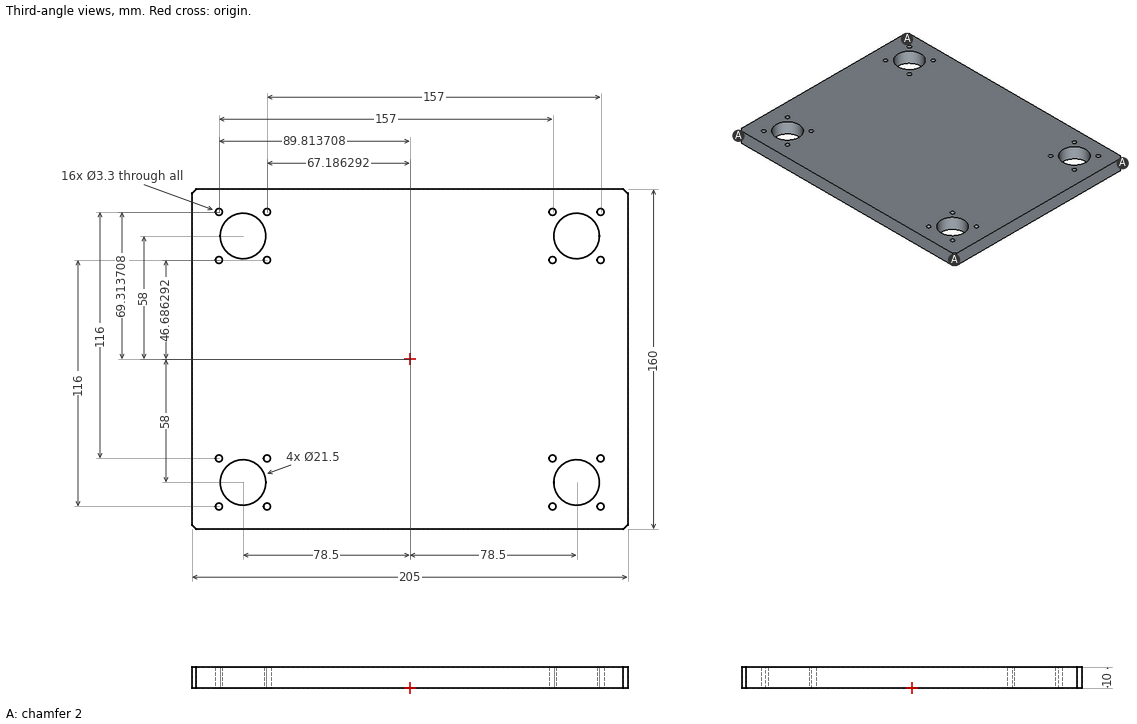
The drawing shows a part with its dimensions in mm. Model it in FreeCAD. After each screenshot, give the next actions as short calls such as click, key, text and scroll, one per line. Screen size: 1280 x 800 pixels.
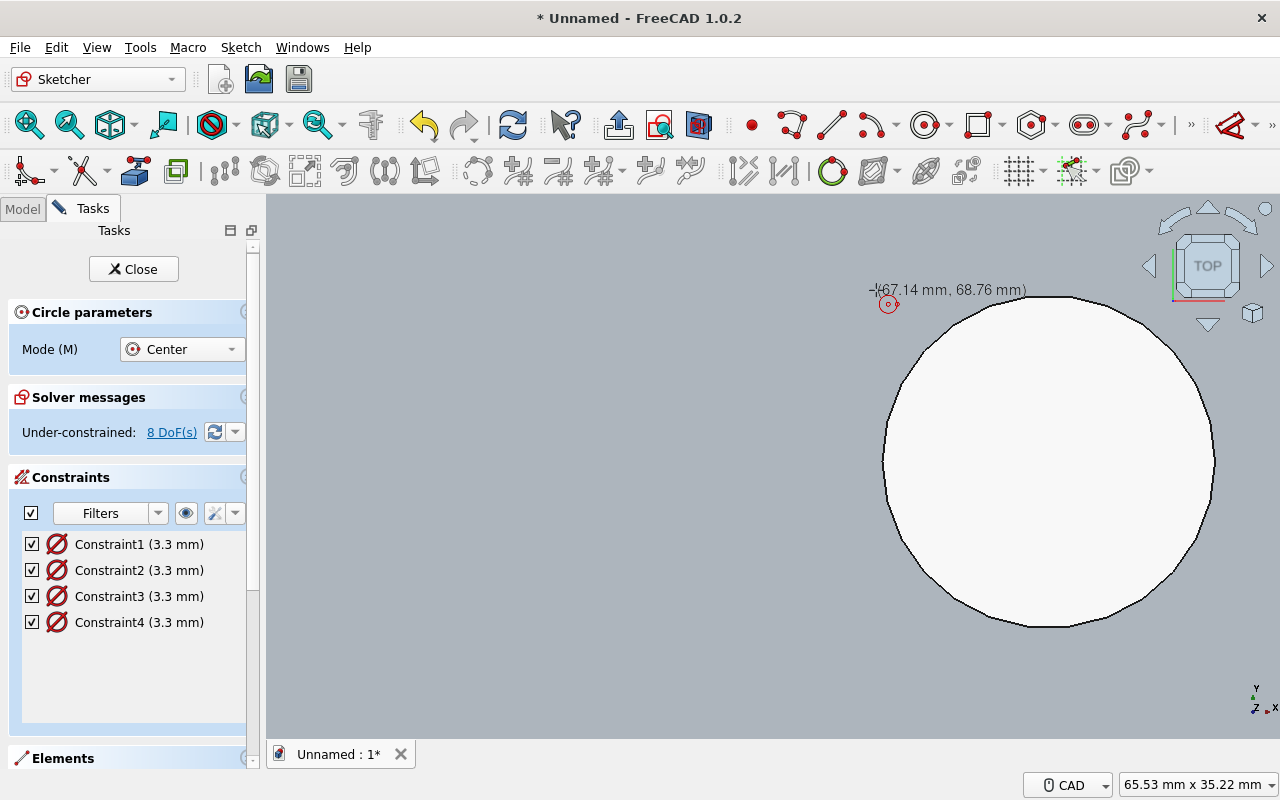
scroll(877, 290, down, 9)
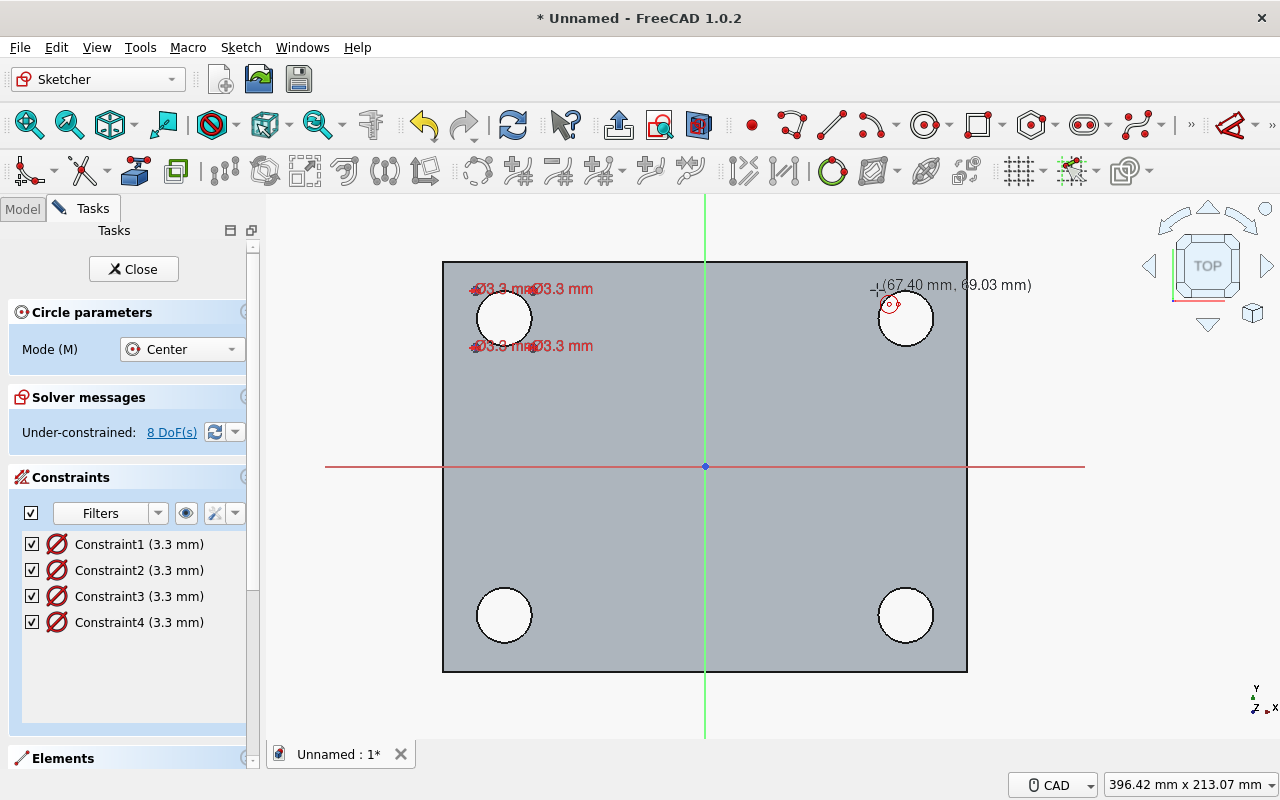
click(877, 290)
move(880, 287)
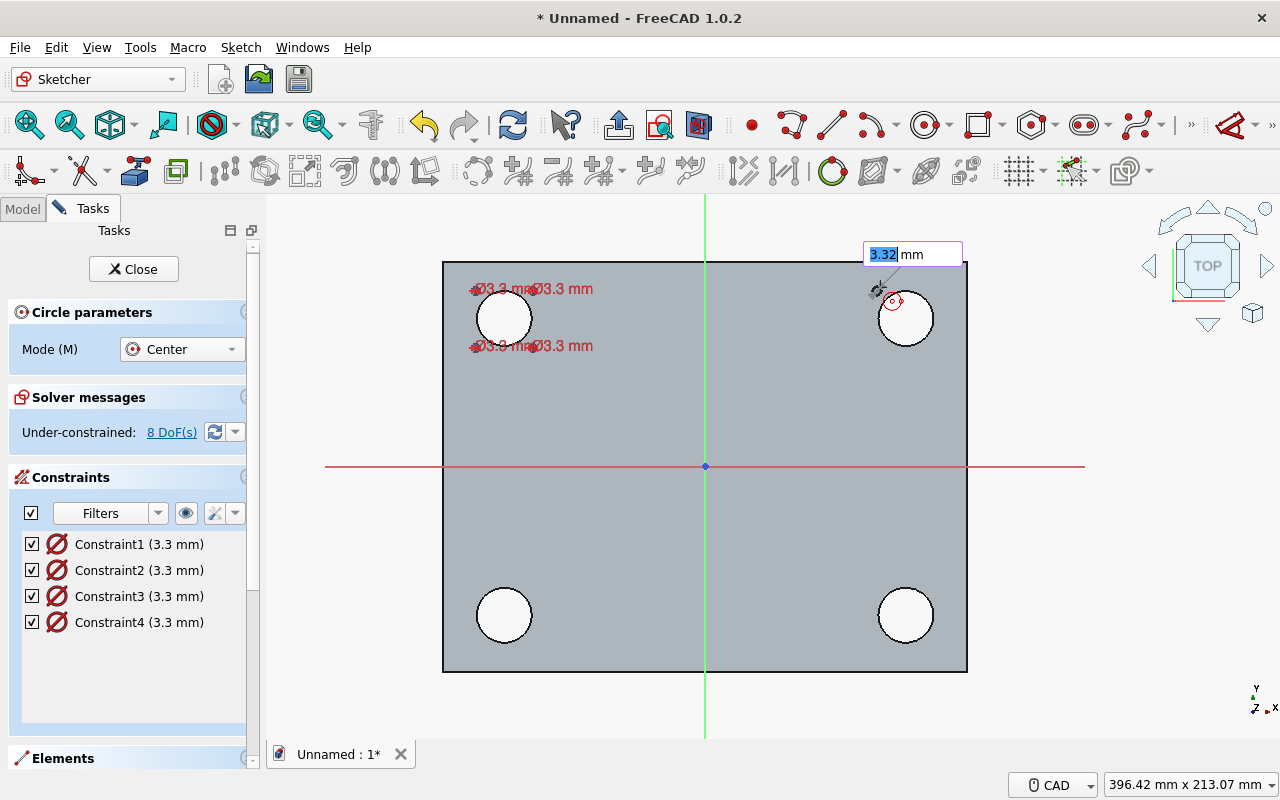
text(3.3)
key(Return)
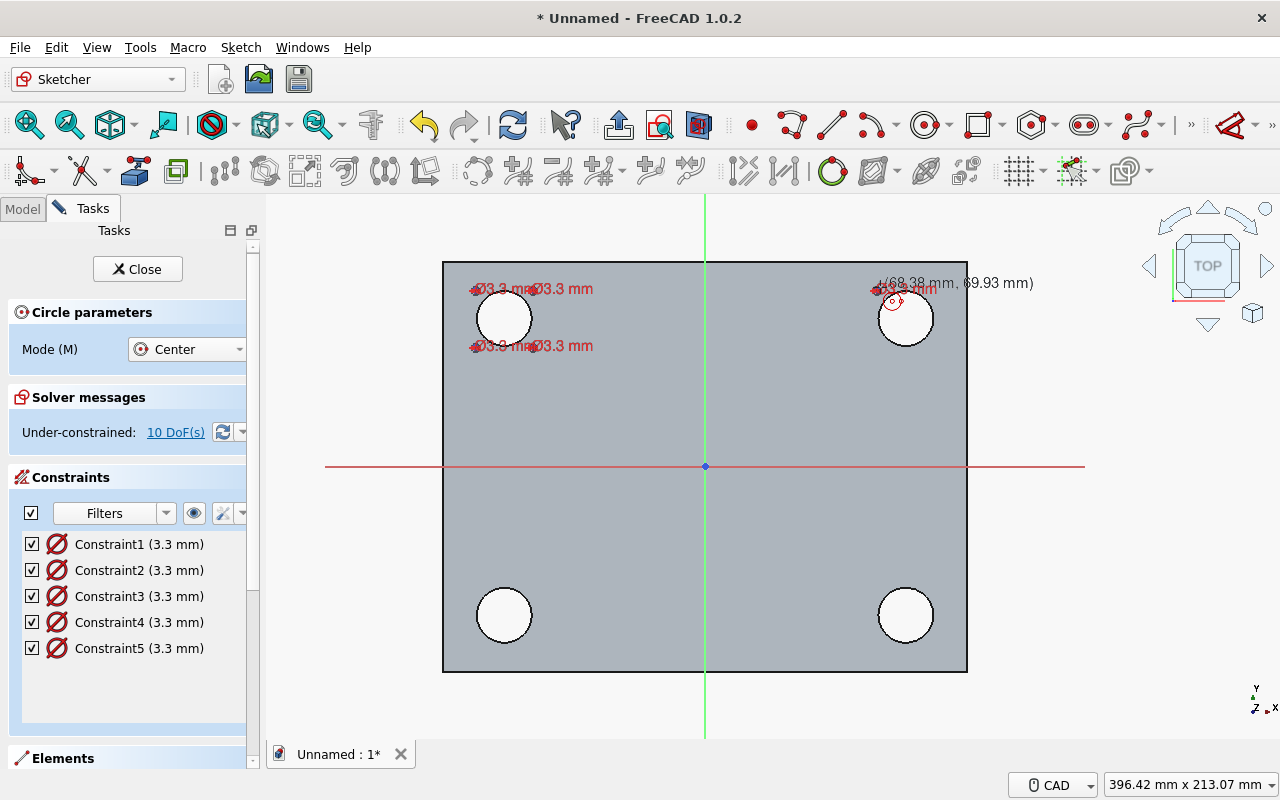
scroll(935, 290, up, 9)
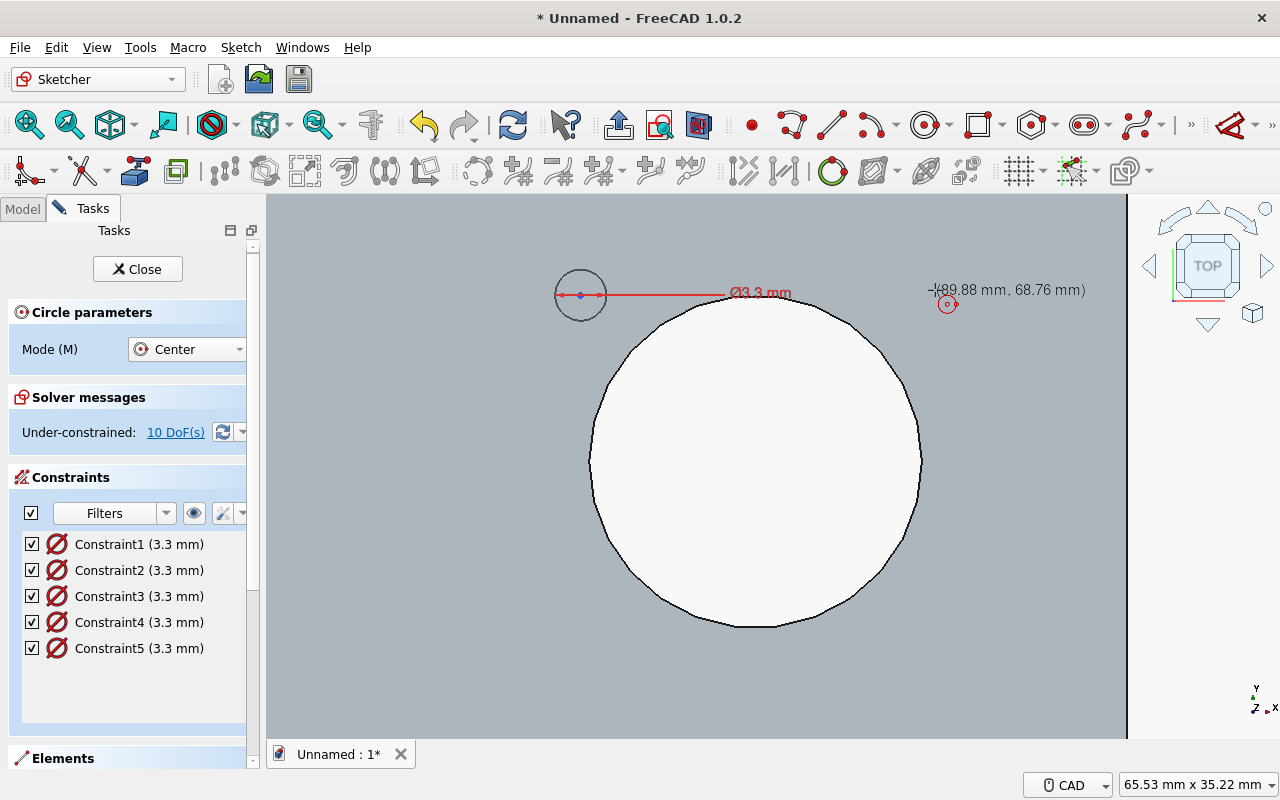
scroll(935, 290, down, 9)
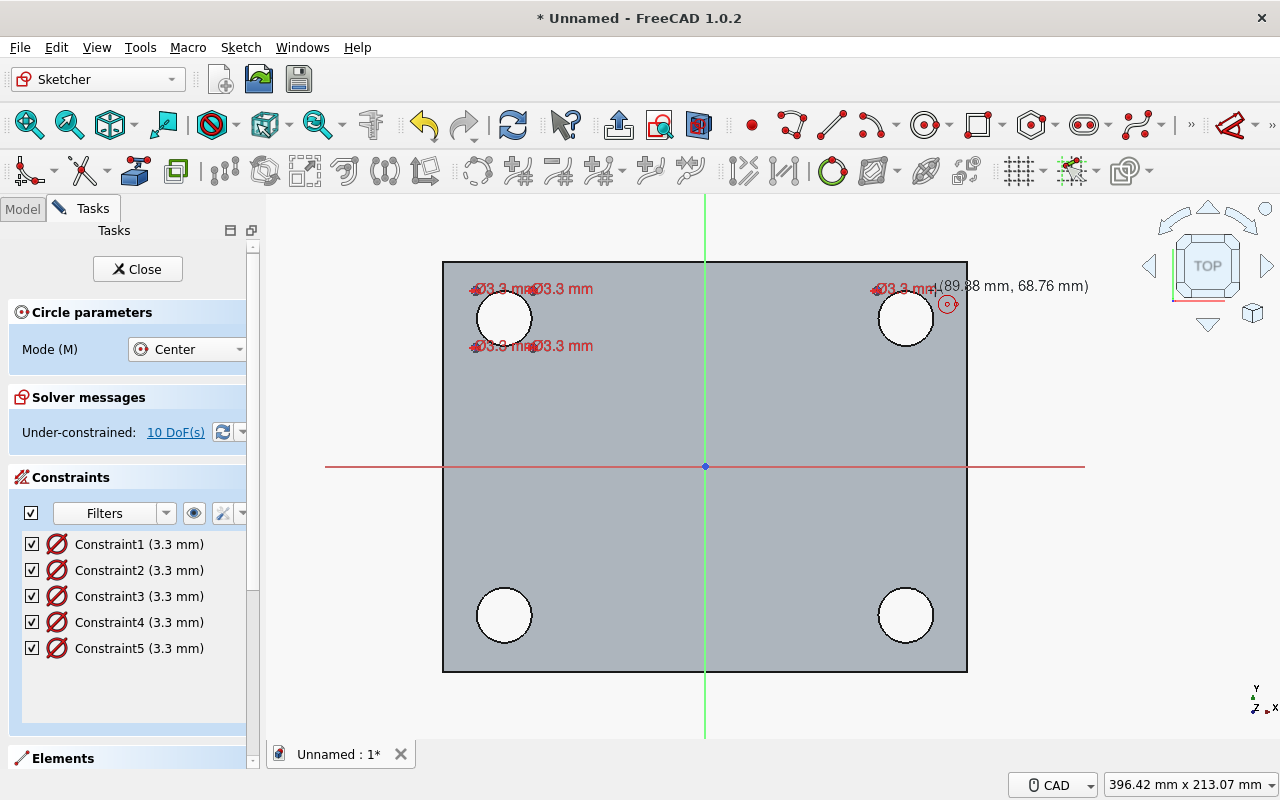
click(935, 290)
move(938, 287)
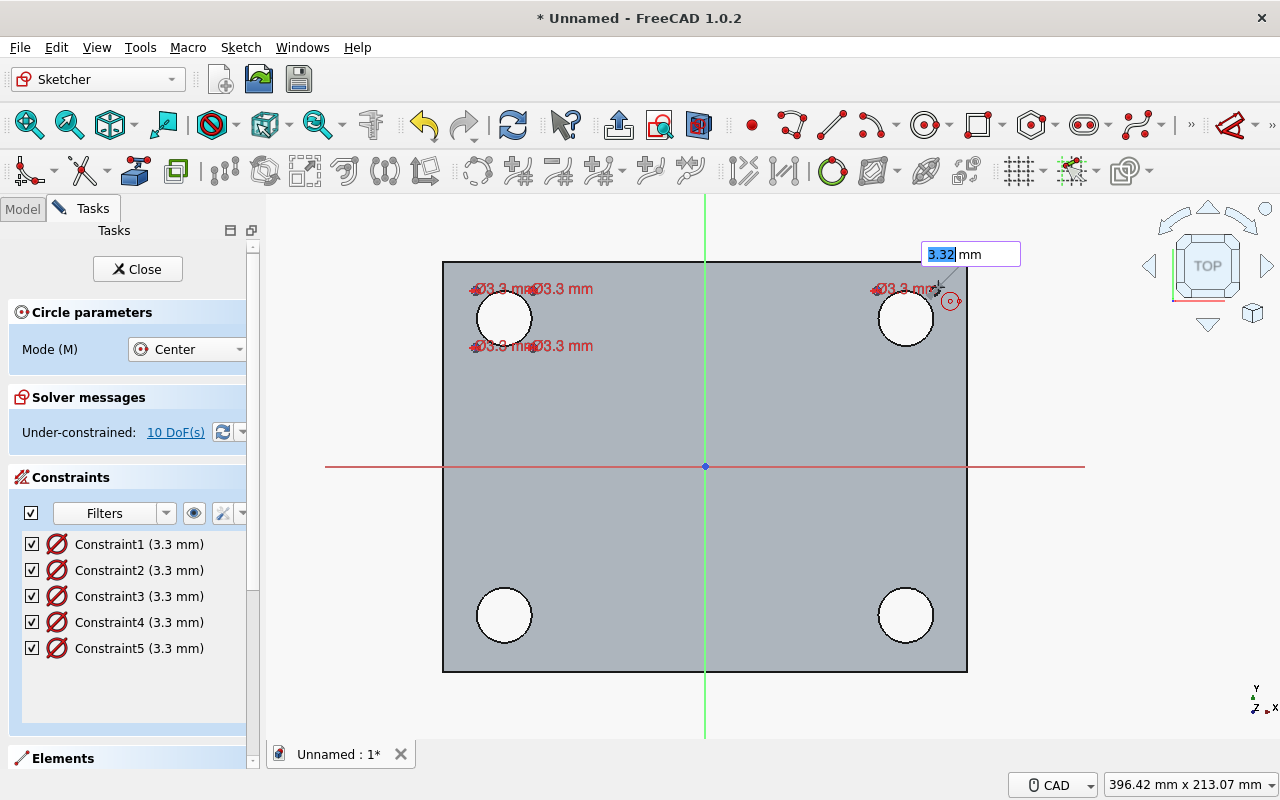
text(3.3)
key(Return)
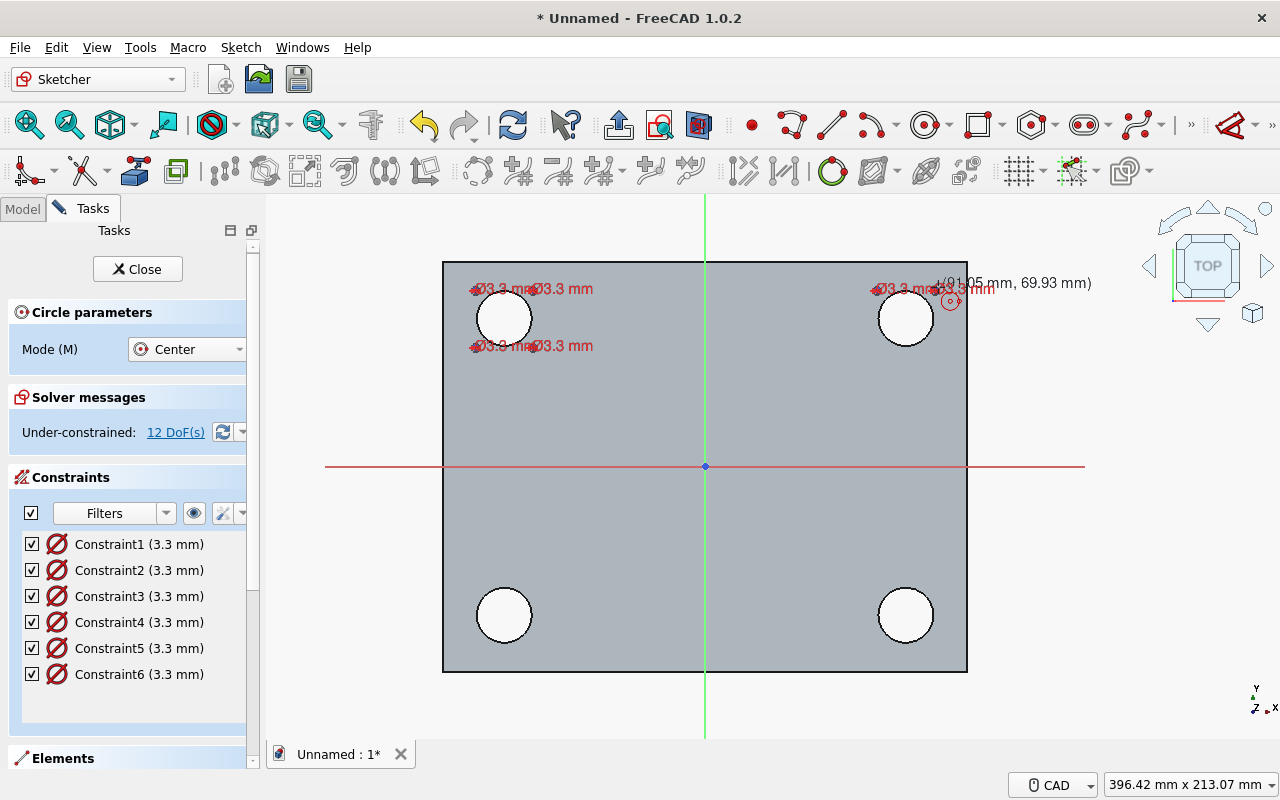
scroll(877, 347, up, 9)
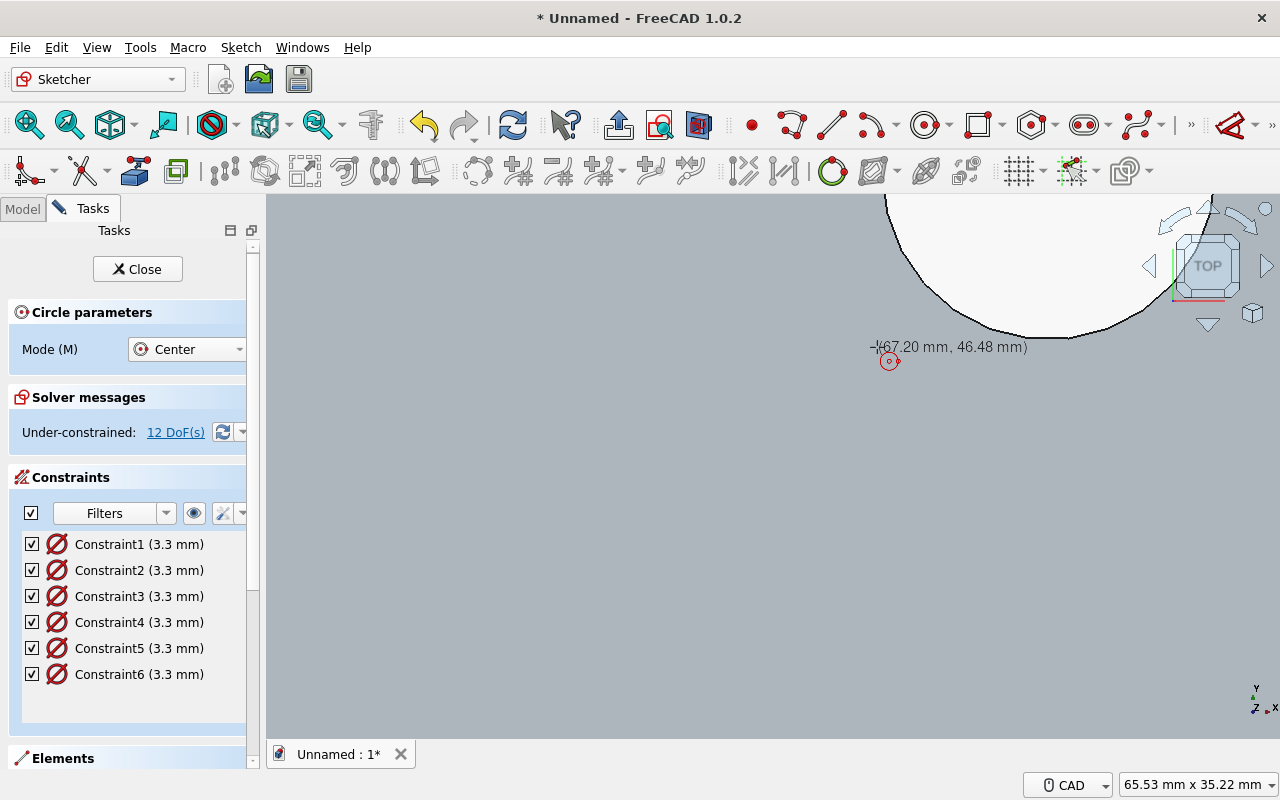
scroll(877, 347, down, 9)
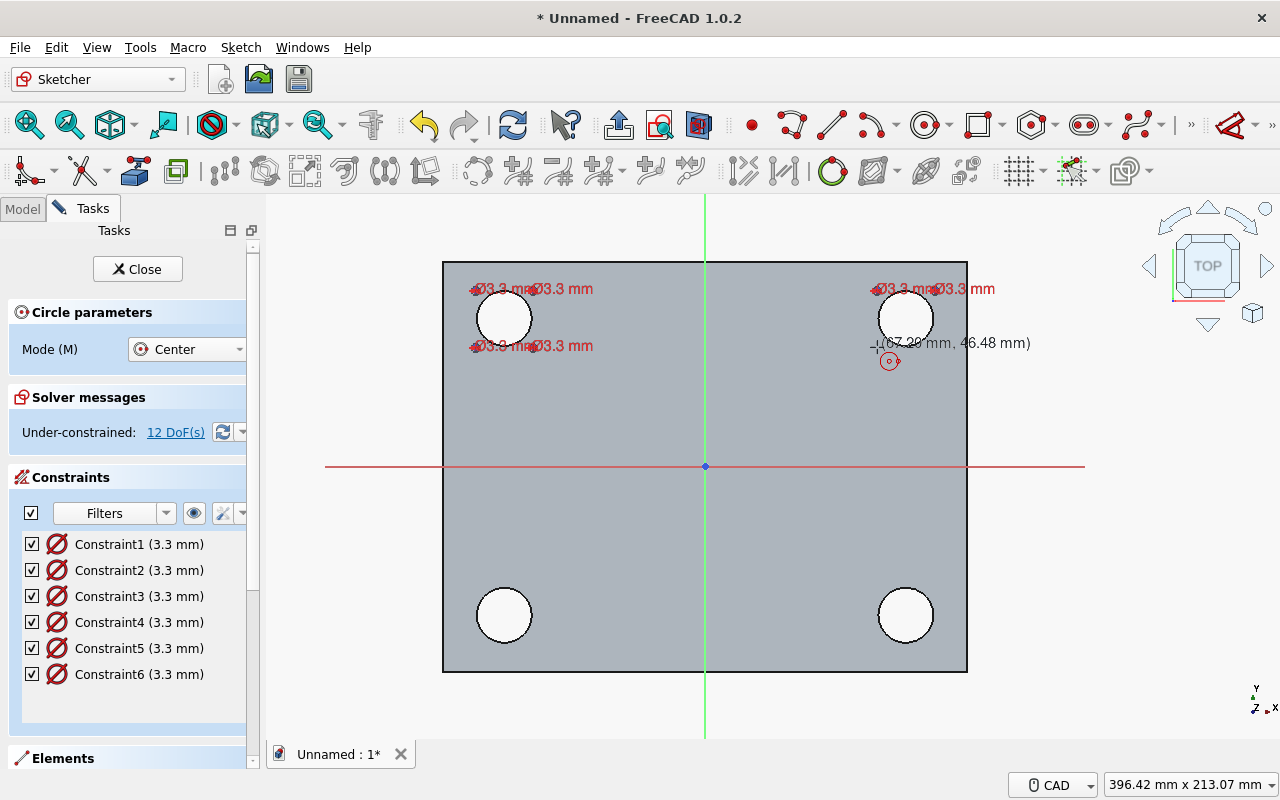
click(877, 347)
move(880, 344)